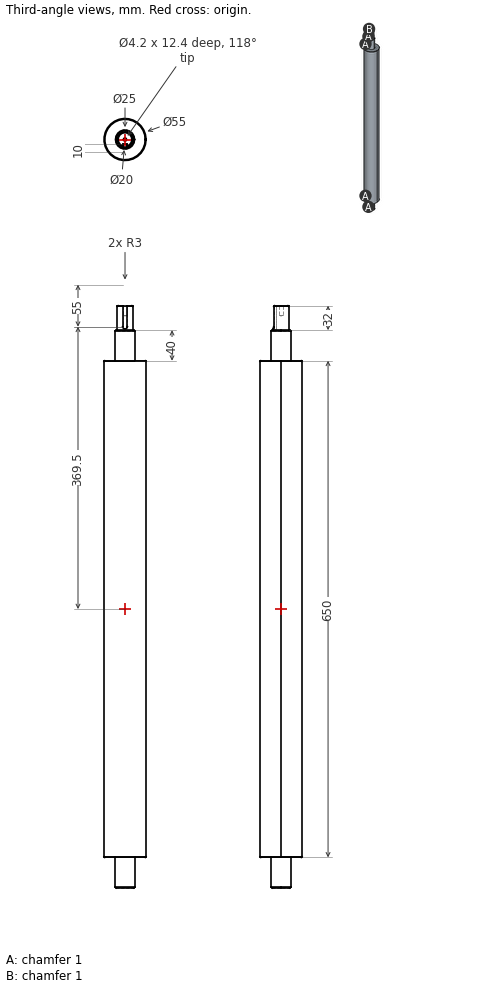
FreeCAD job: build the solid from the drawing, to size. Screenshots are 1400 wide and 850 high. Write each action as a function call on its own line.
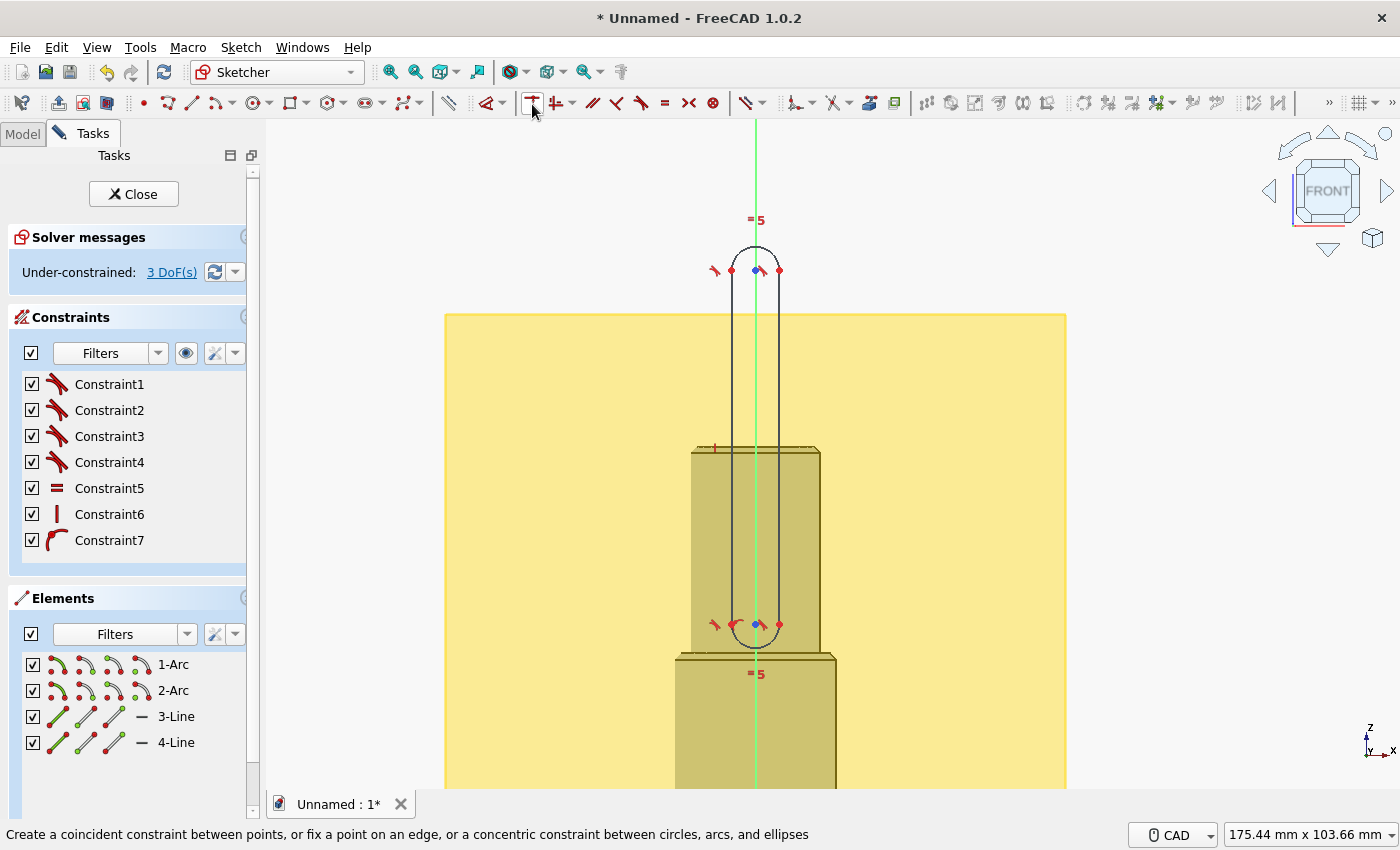
click(486, 104)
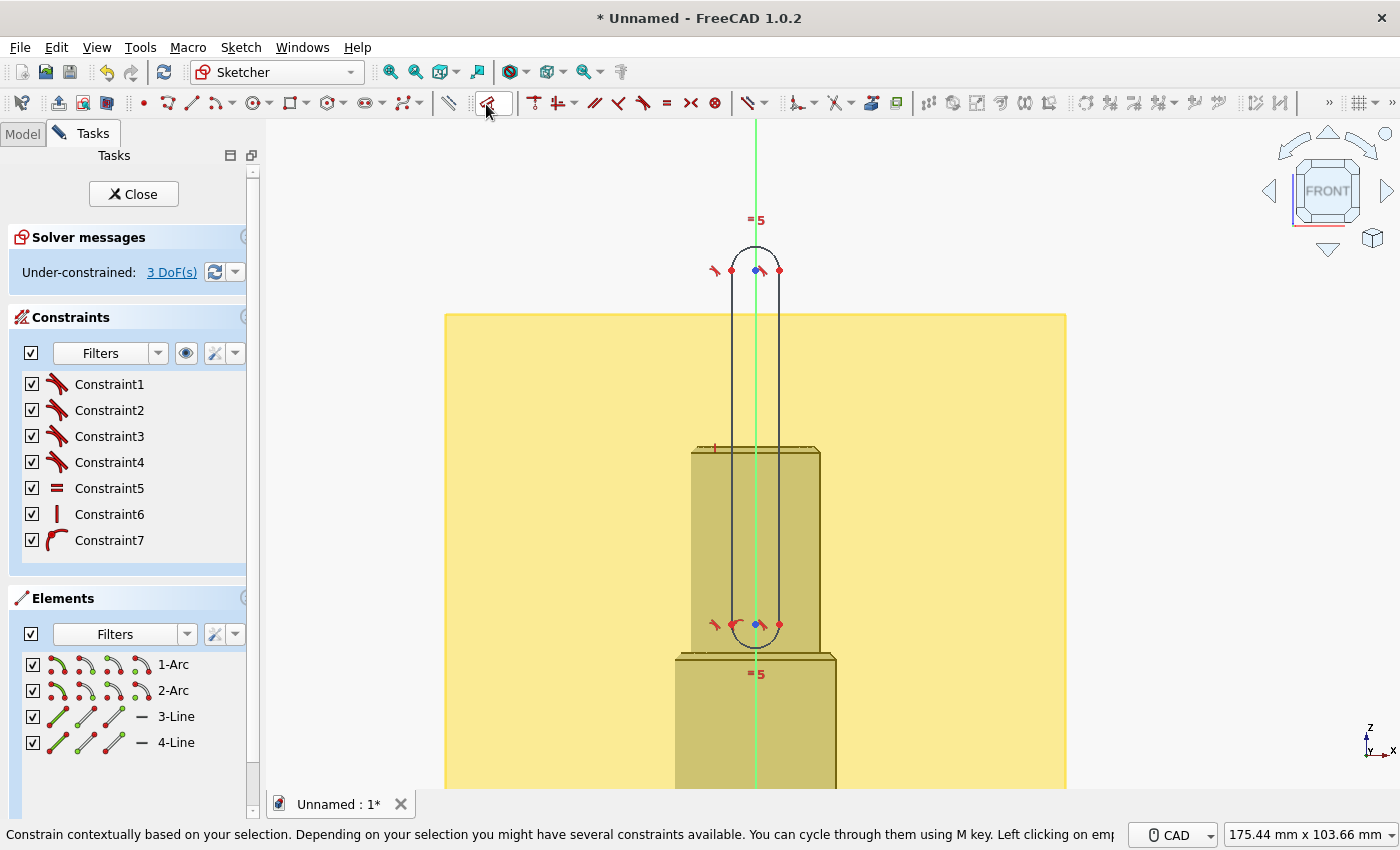
scroll(742, 644, up, 4)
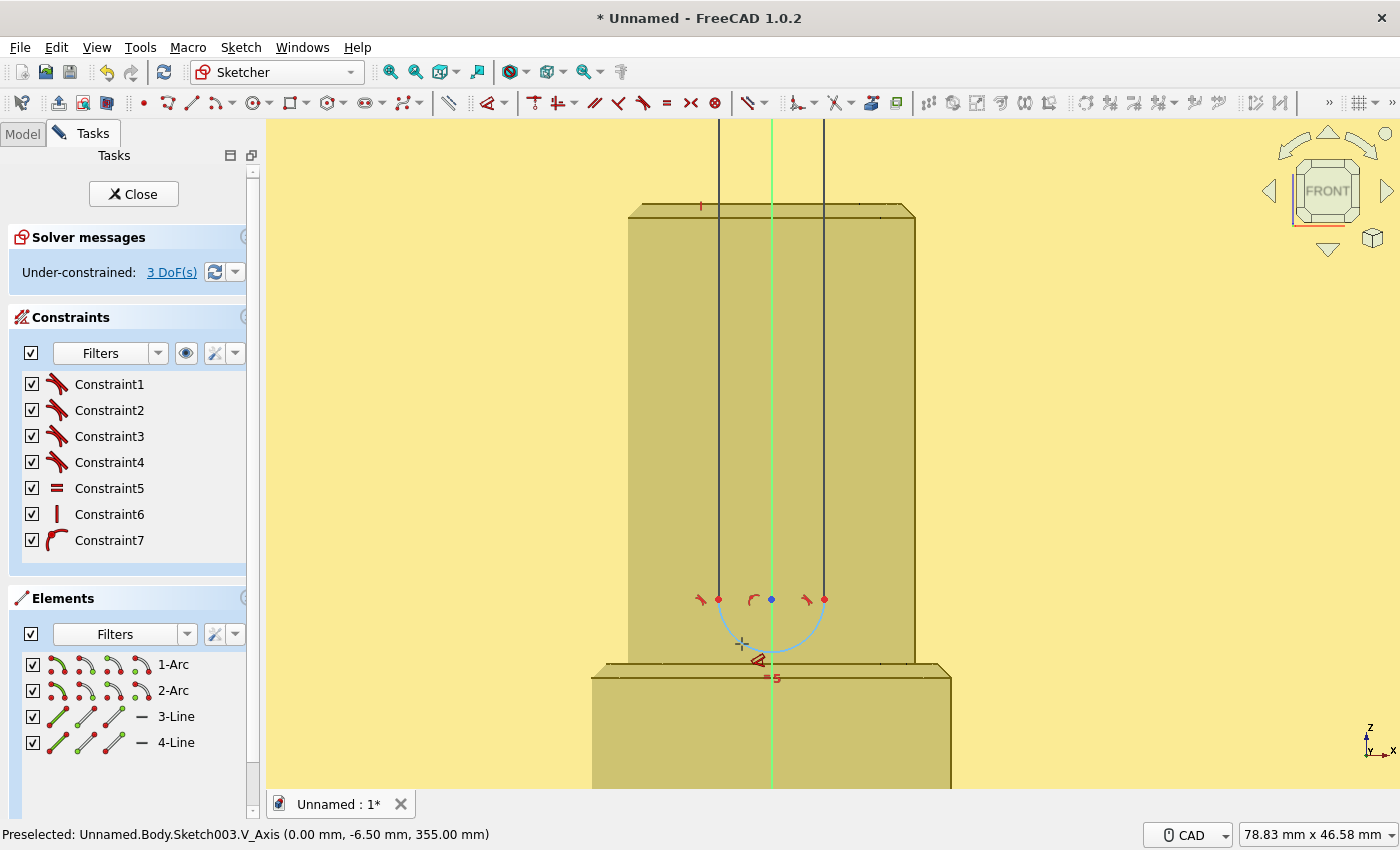
click(740, 642)
click(721, 668)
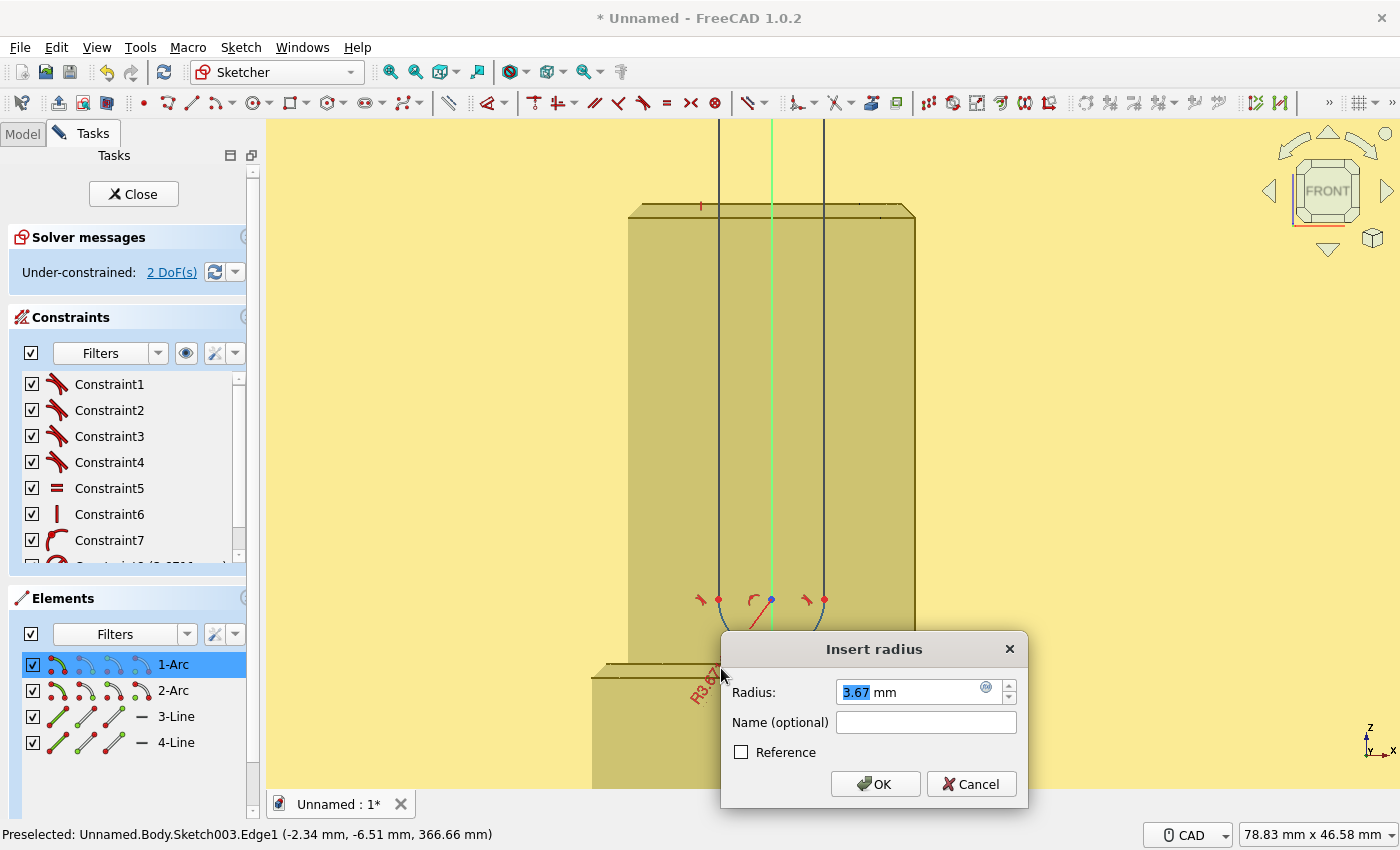
text(3)
key(Return)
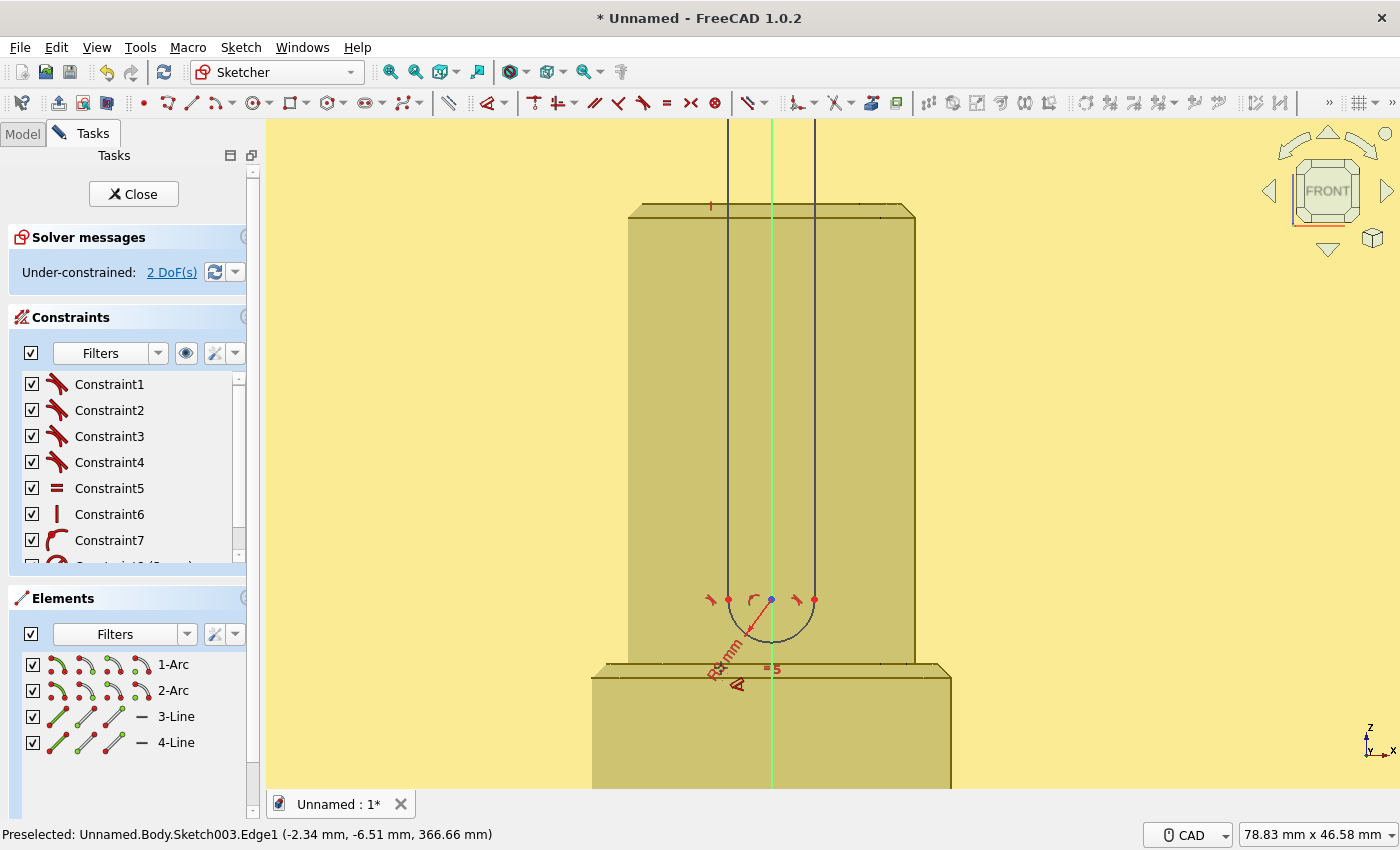
click(728, 363)
click(694, 373)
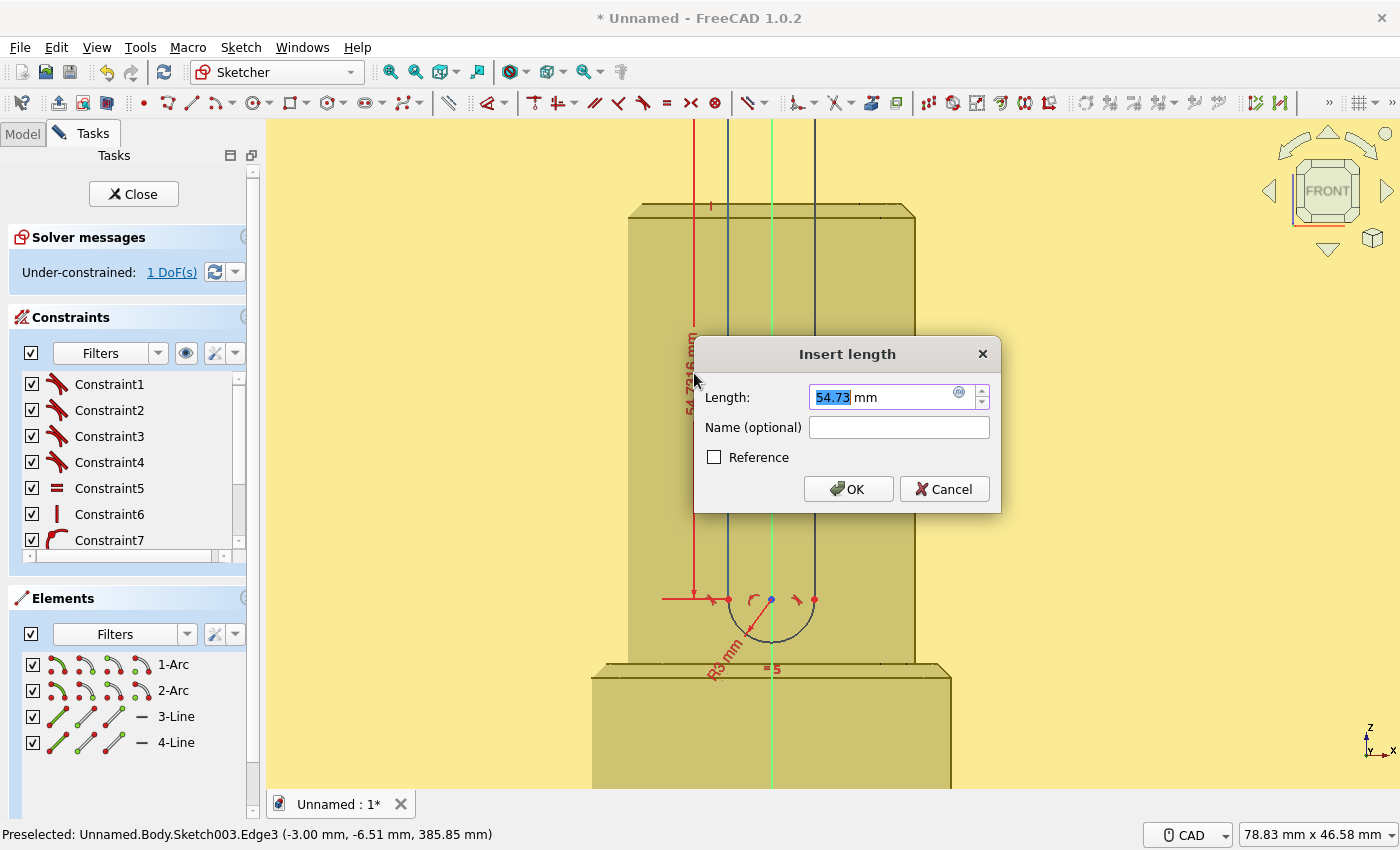
text(55)
key(Return)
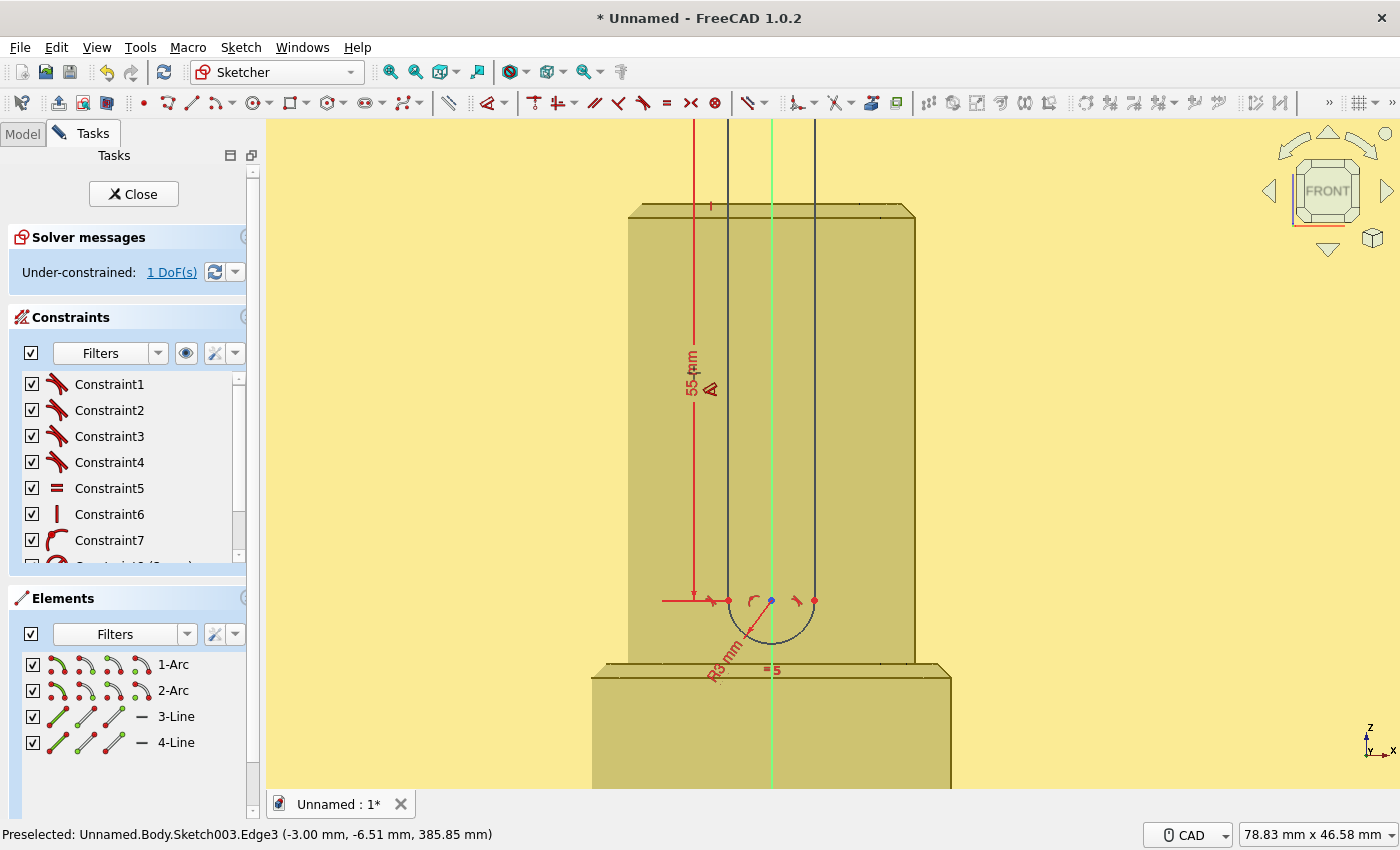
click(728, 601)
click(694, 644)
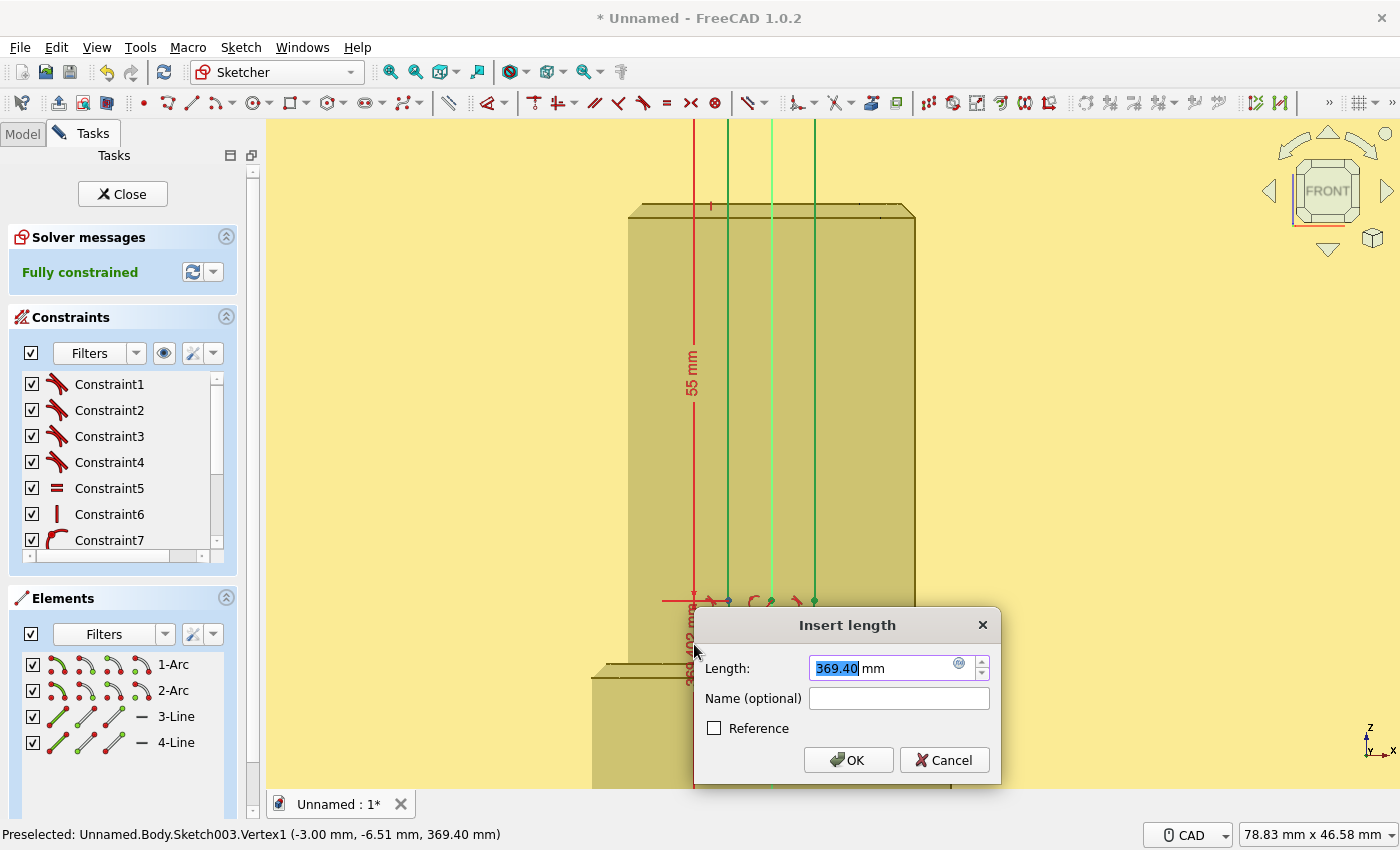
text(369.5)
key(Return)
key(Escape)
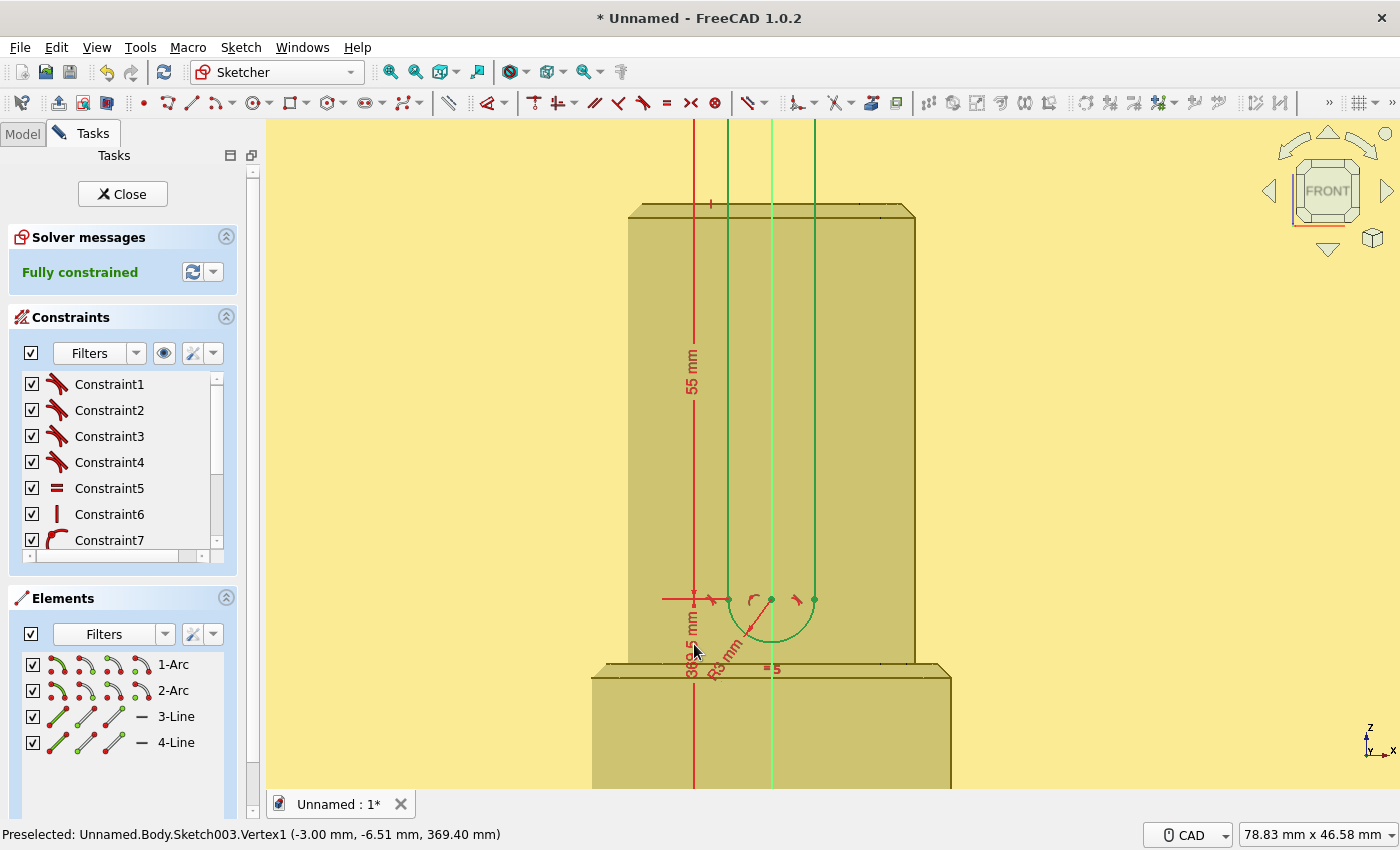
click(123, 194)